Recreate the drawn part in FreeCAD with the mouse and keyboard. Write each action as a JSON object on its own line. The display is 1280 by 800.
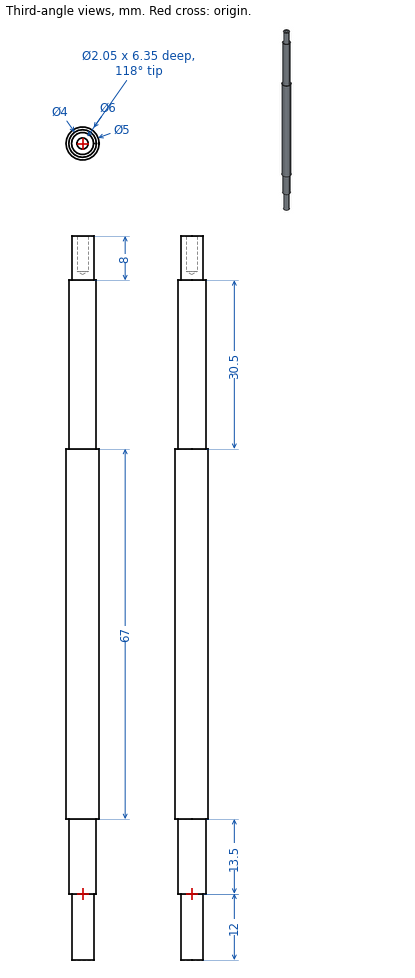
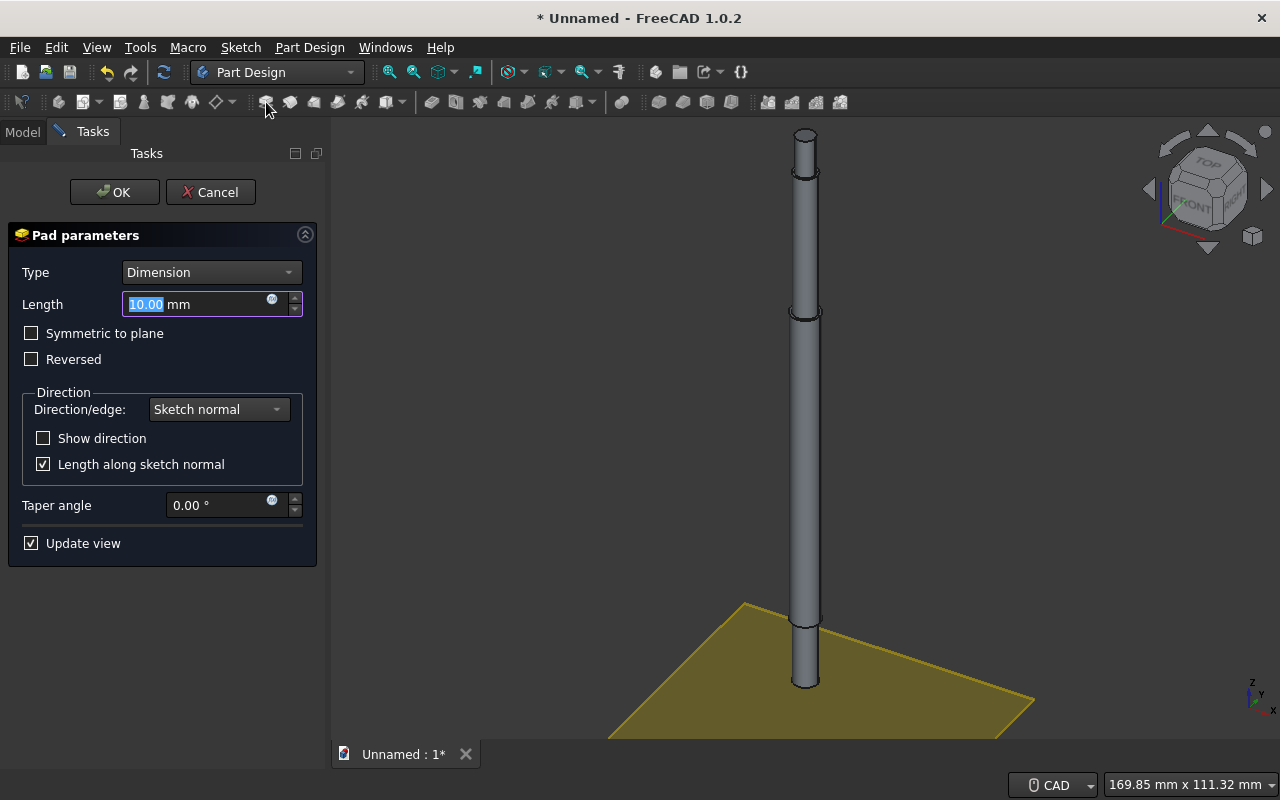
{"action": "type", "text": "12"}
{"action": "key", "text": "Tab"}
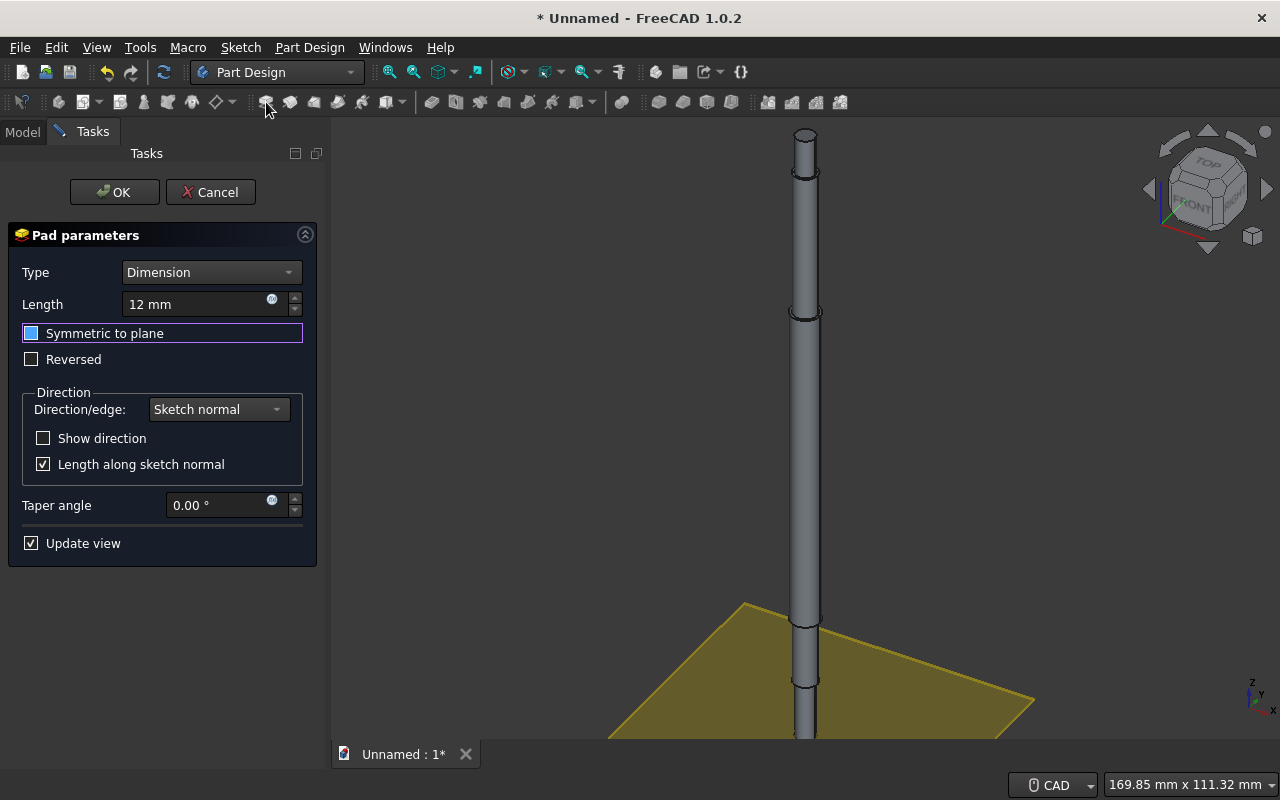
{"action": "left_click", "coordinate": [115, 192]}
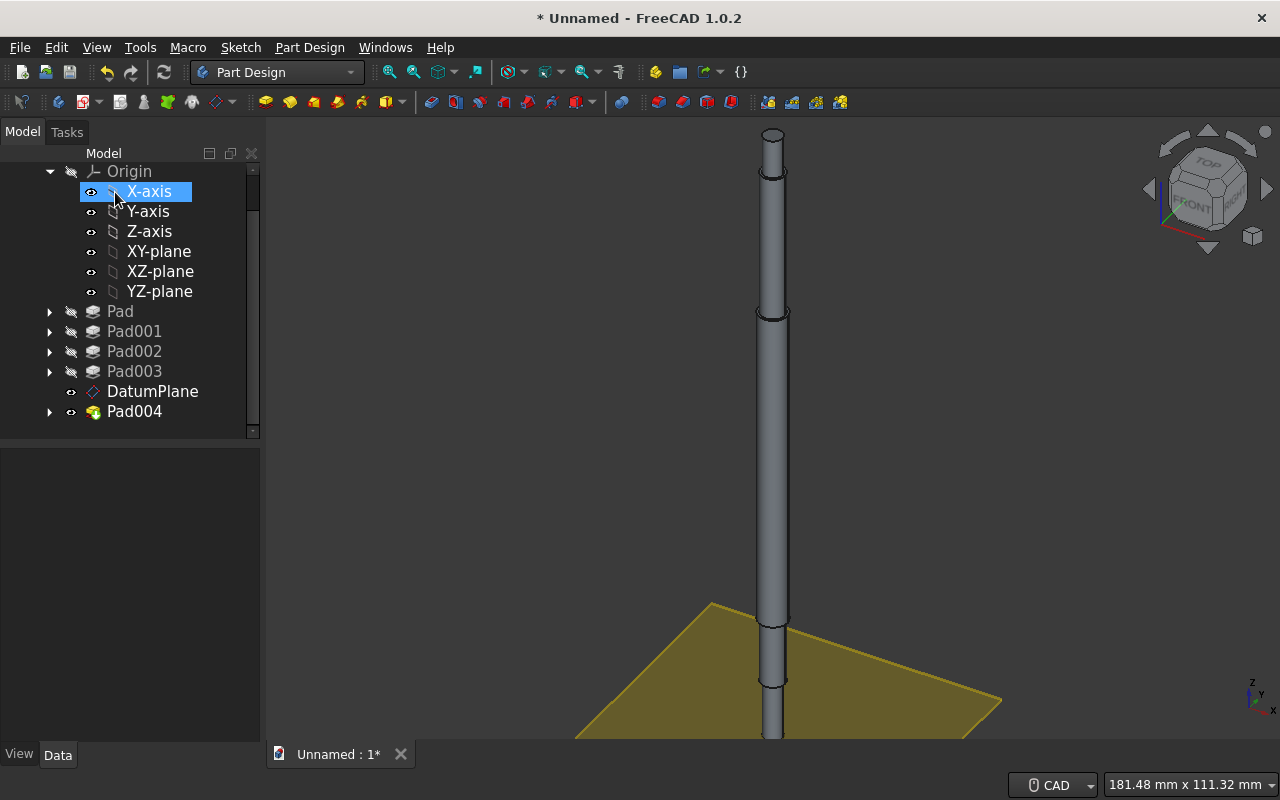
{"action": "left_click", "coordinate": [116, 392]}
{"action": "key", "text": "space"}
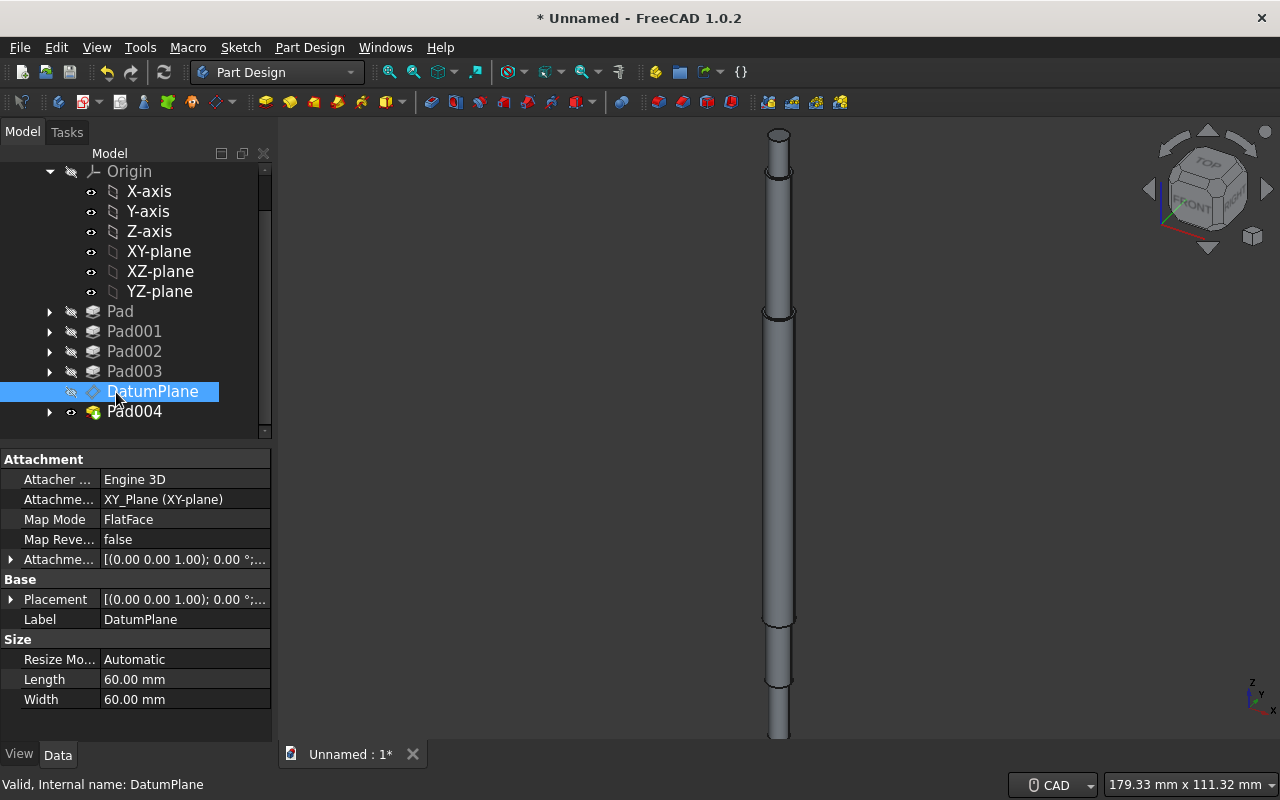
{"action": "left_click", "coordinate": [390, 72]}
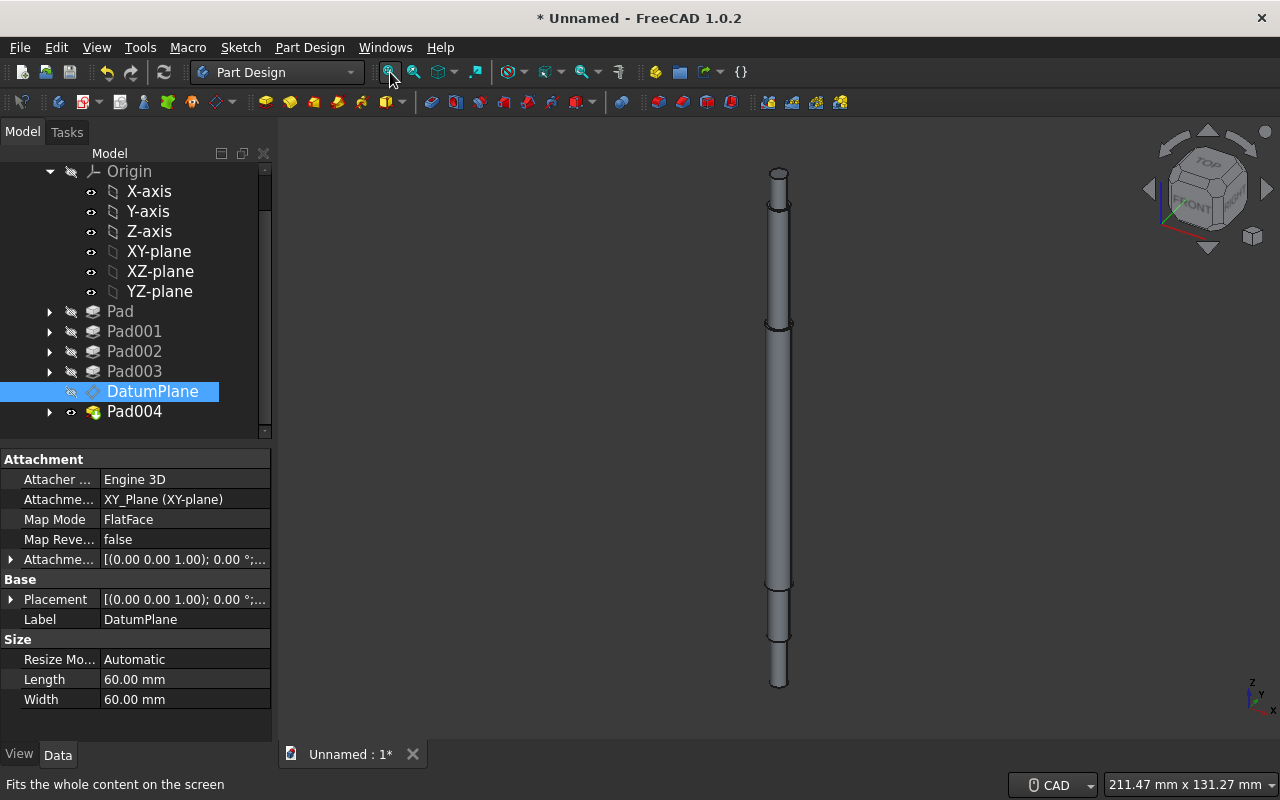
{"action": "key", "text": "0"}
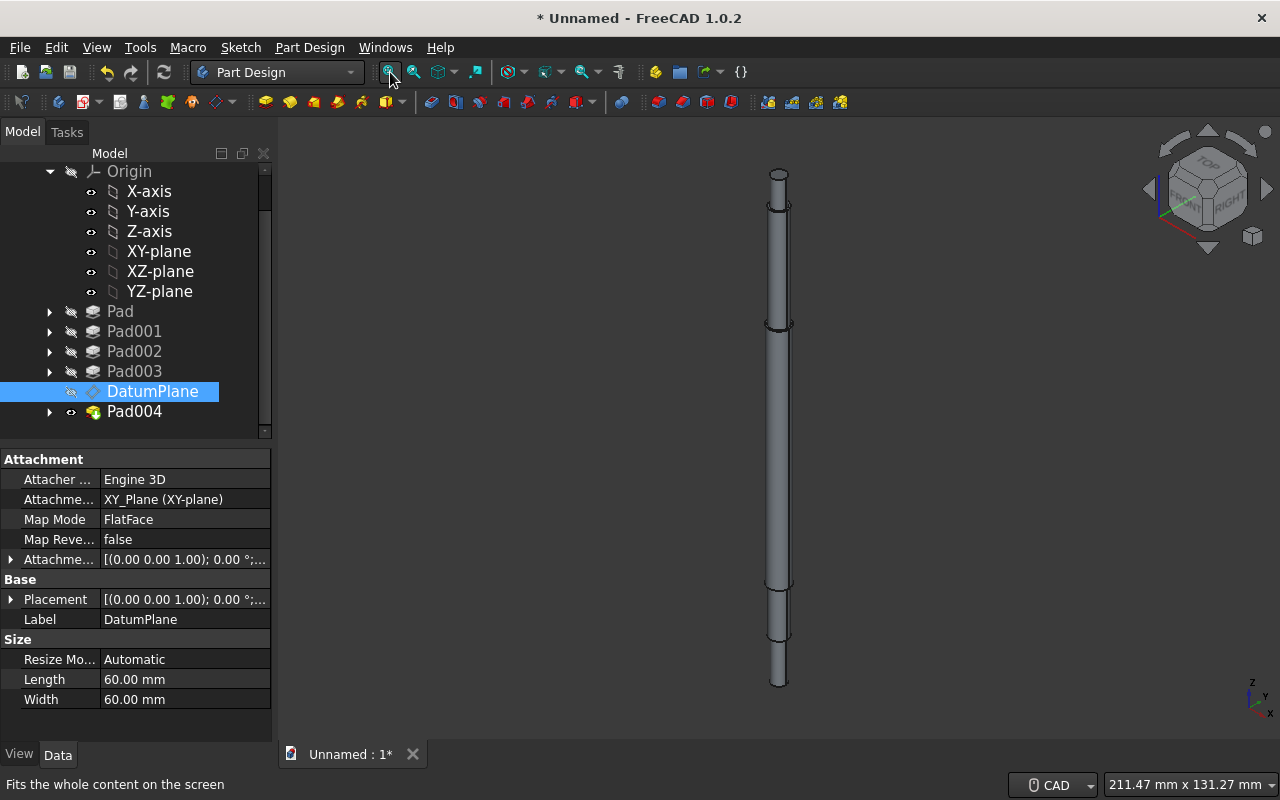
{"action": "key", "text": "2"}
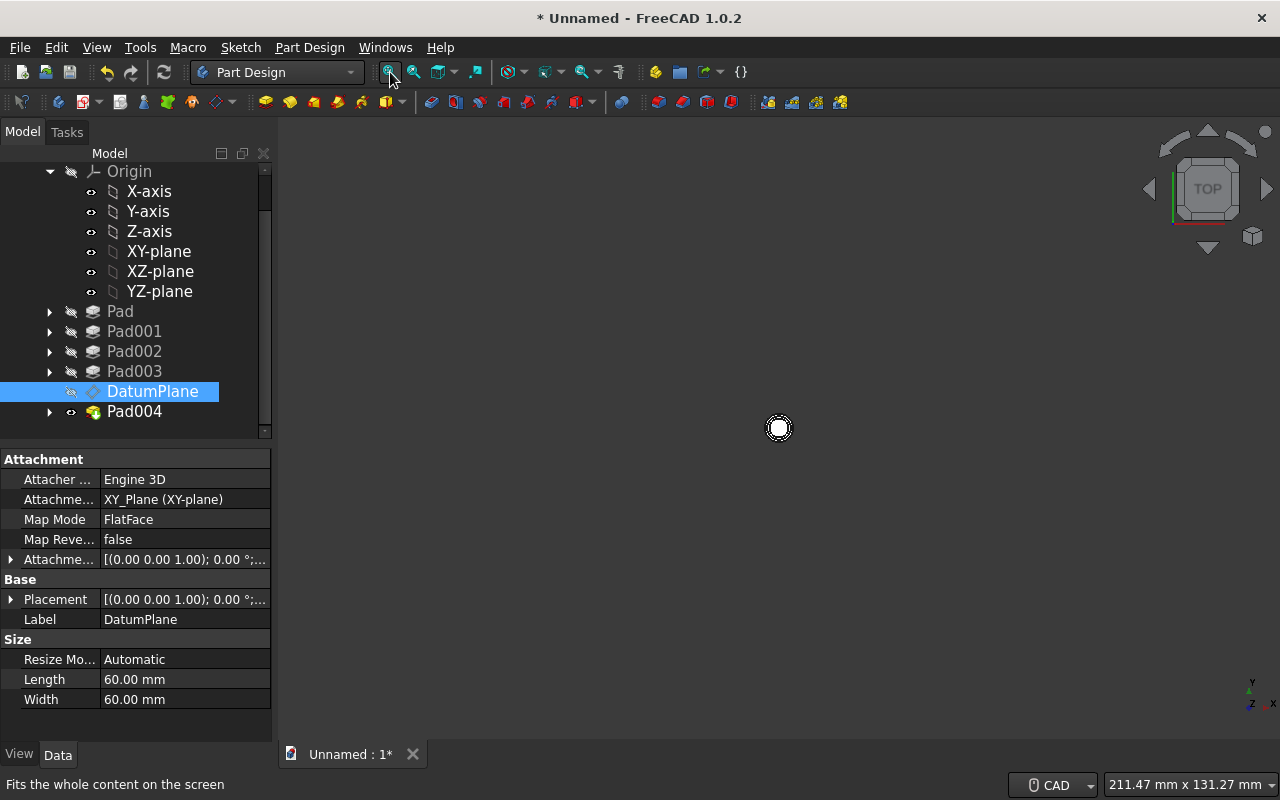
{"action": "left_click", "coordinate": [390, 72]}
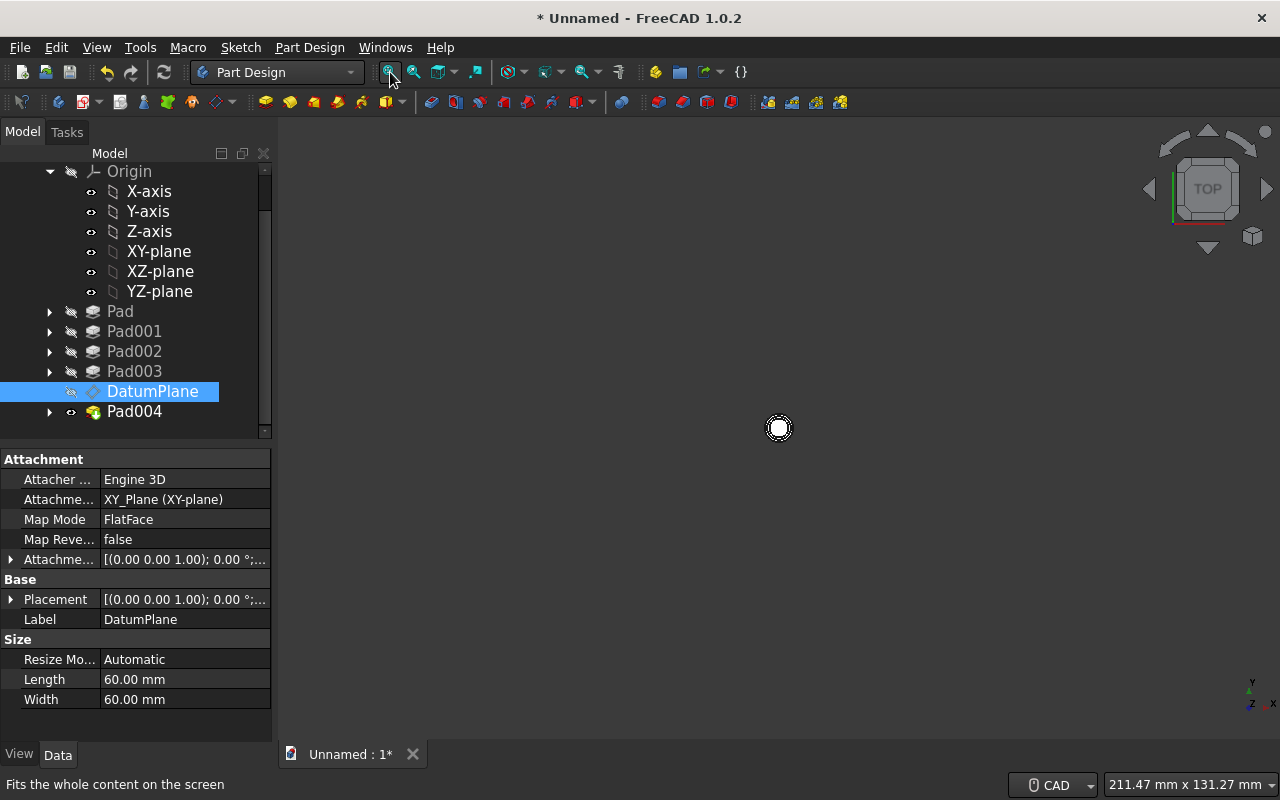
{"action": "left_click", "coordinate": [779, 427]}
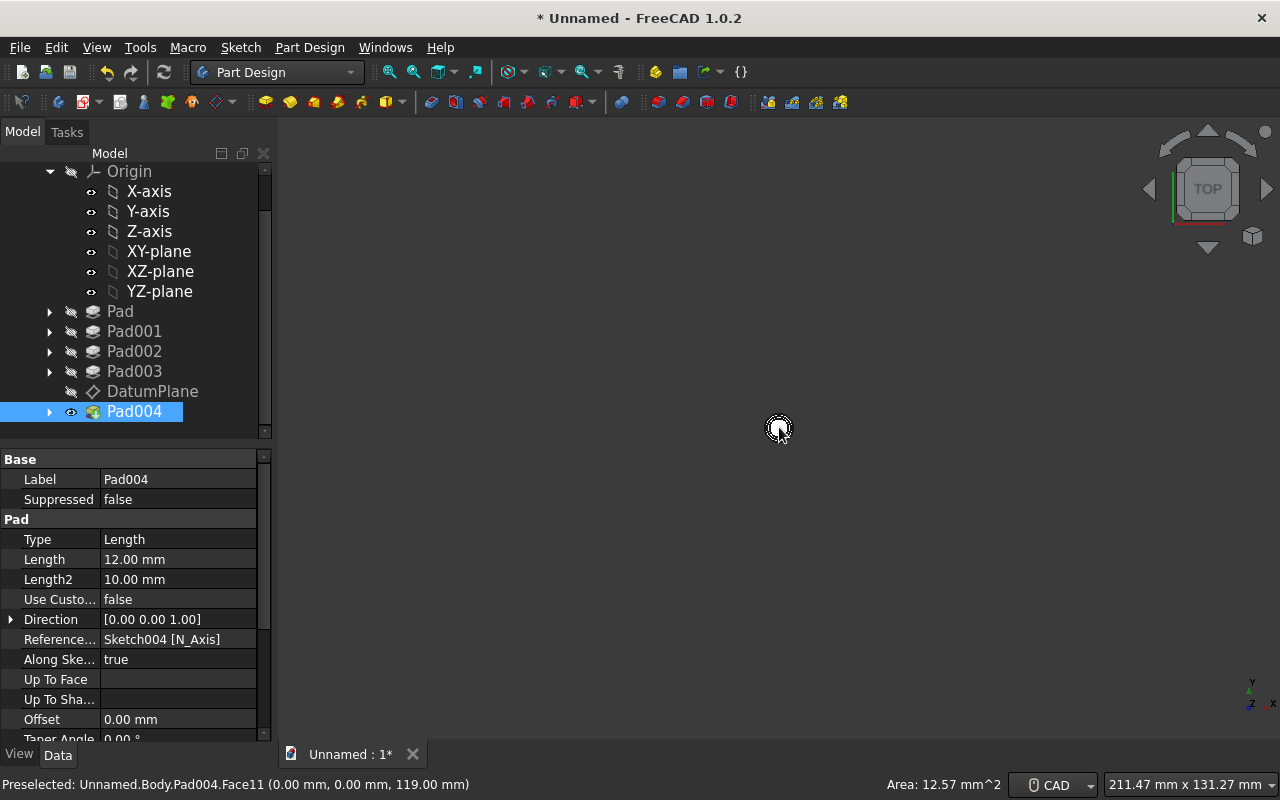
{"action": "left_click", "coordinate": [84, 102]}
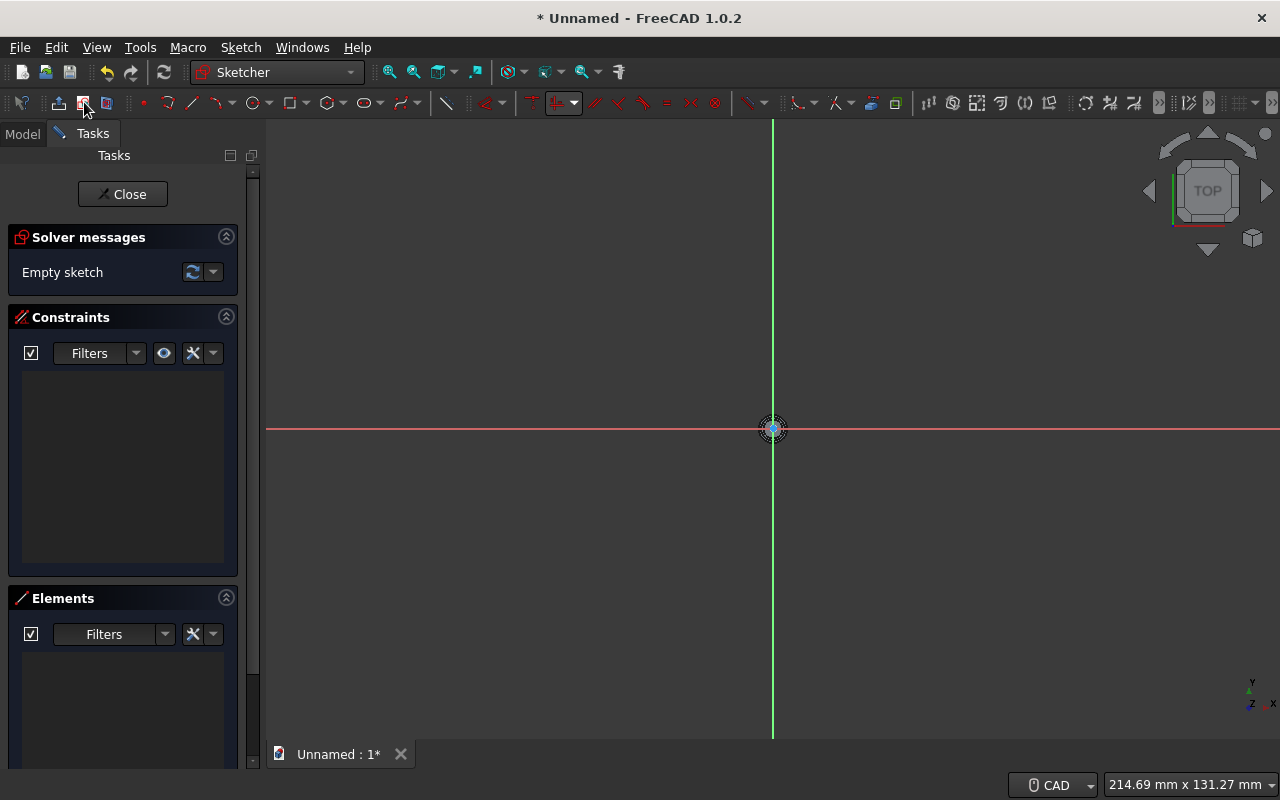
{"action": "scroll", "coordinate": [777, 429], "scroll_direction": "up", "scroll_amount": 15}